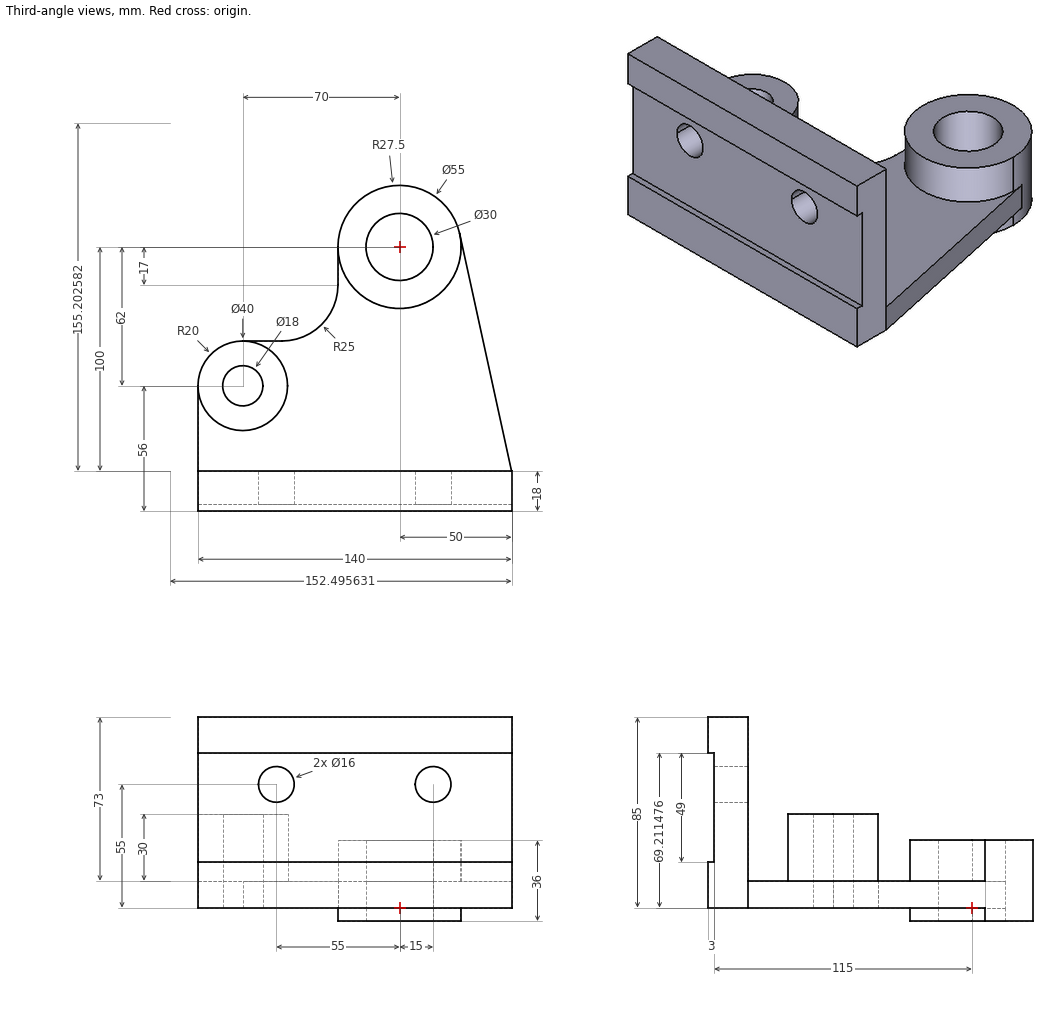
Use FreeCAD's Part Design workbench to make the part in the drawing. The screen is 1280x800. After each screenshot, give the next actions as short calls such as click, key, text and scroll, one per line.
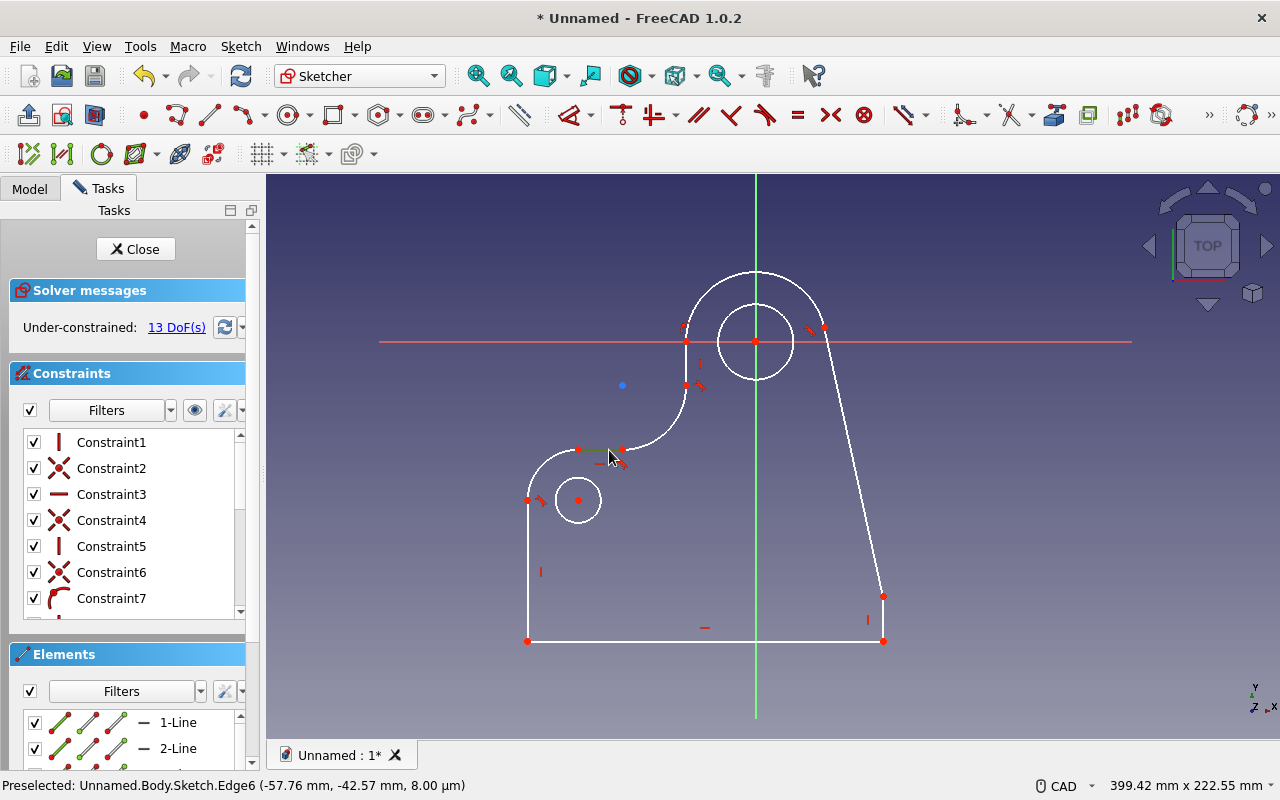
click(555, 455)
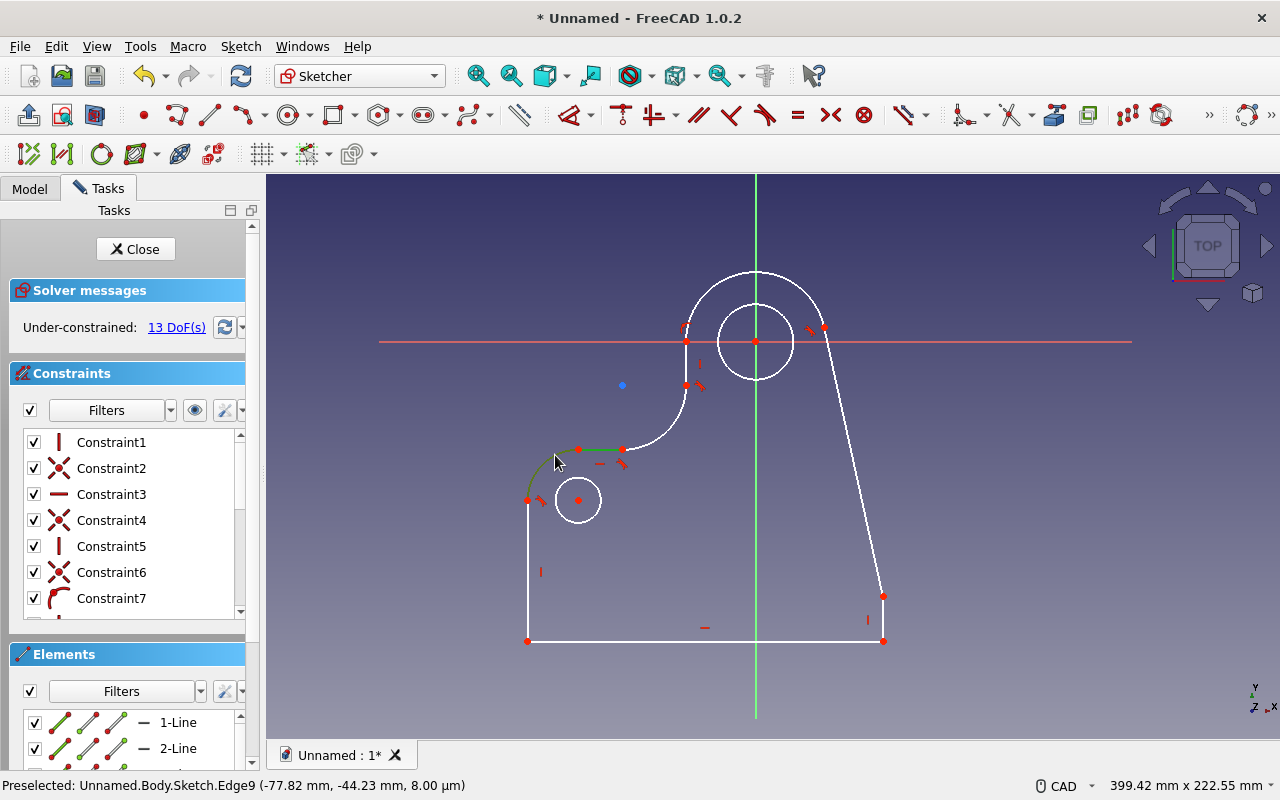
key(t)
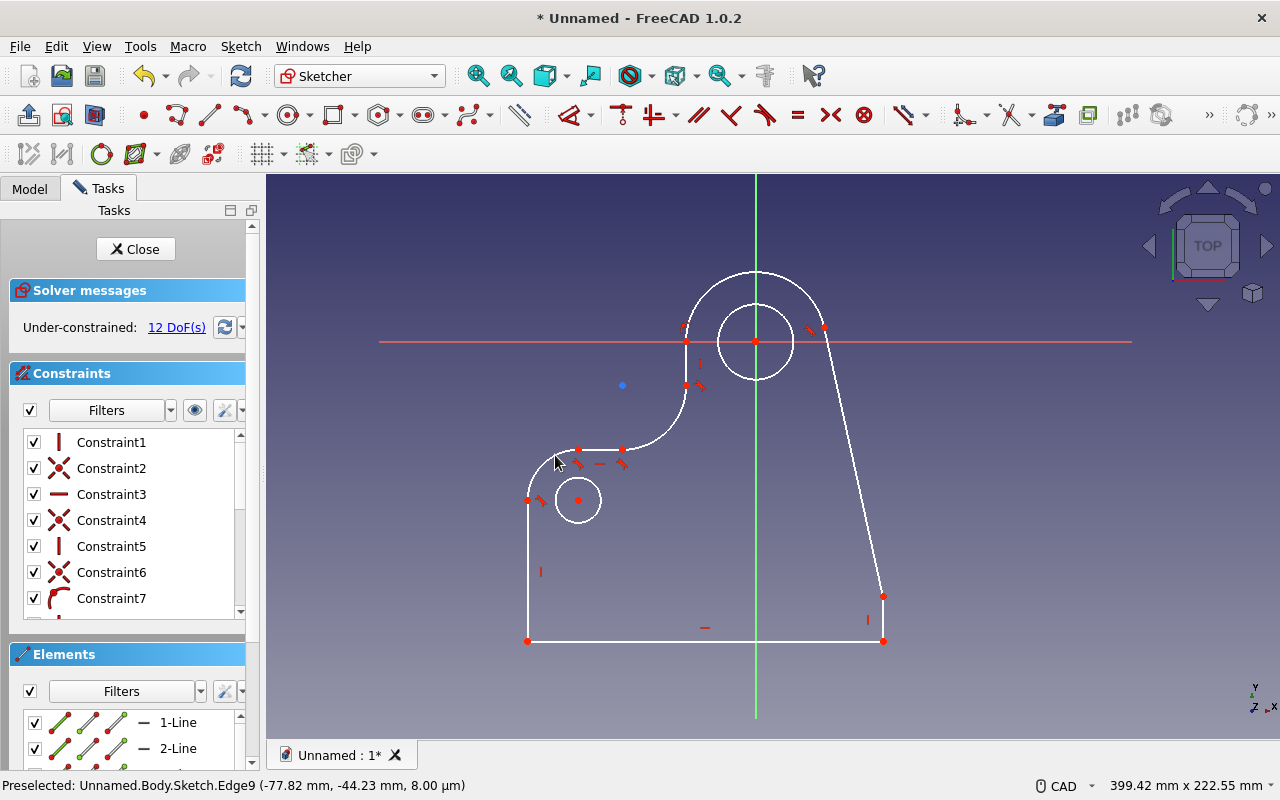
scroll(756, 342, up, 3)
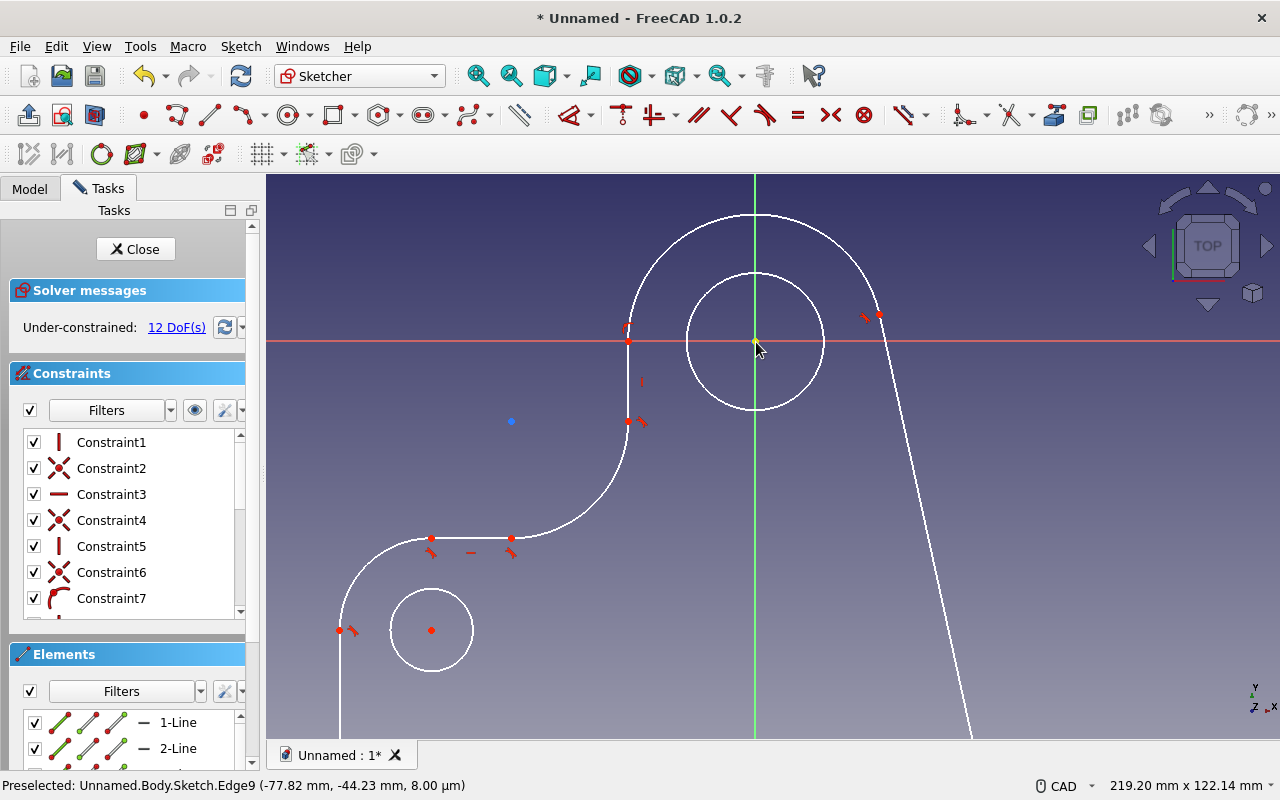
drag(745, 331, 765, 352)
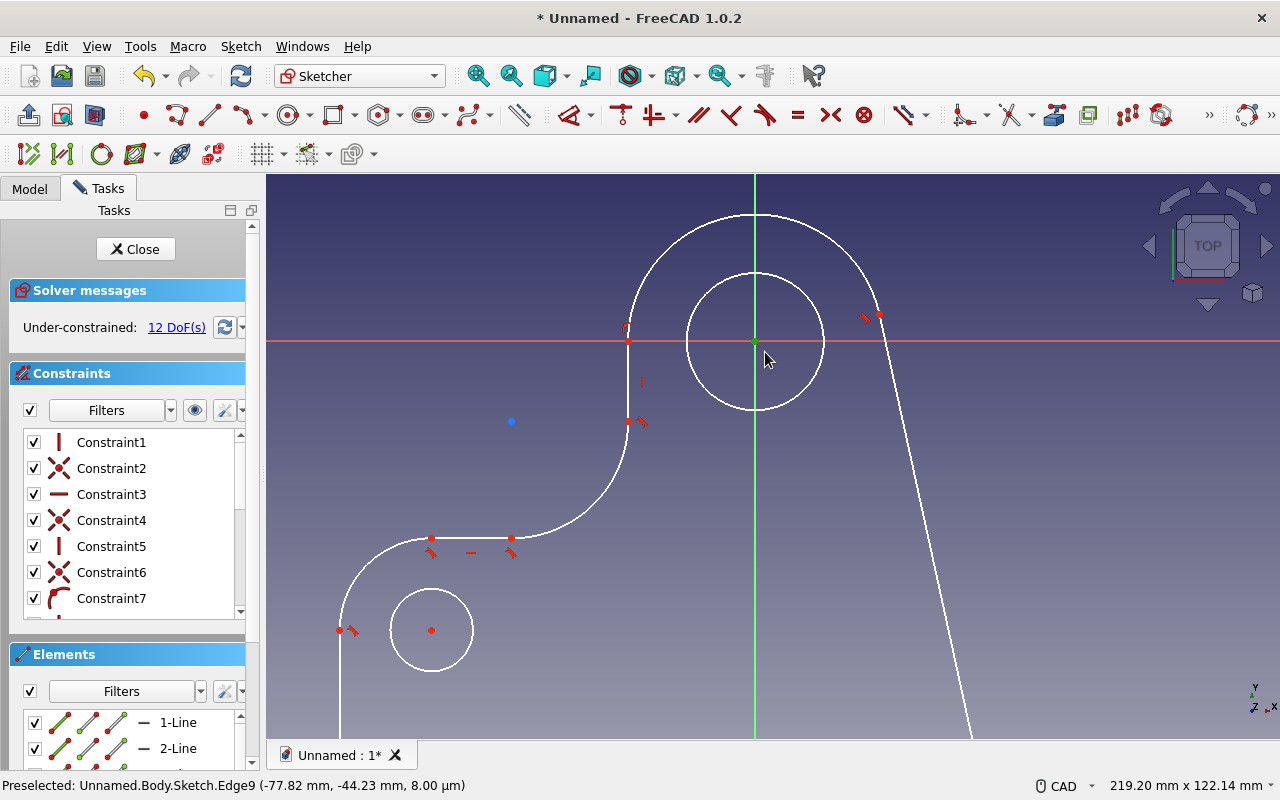
click(621, 116)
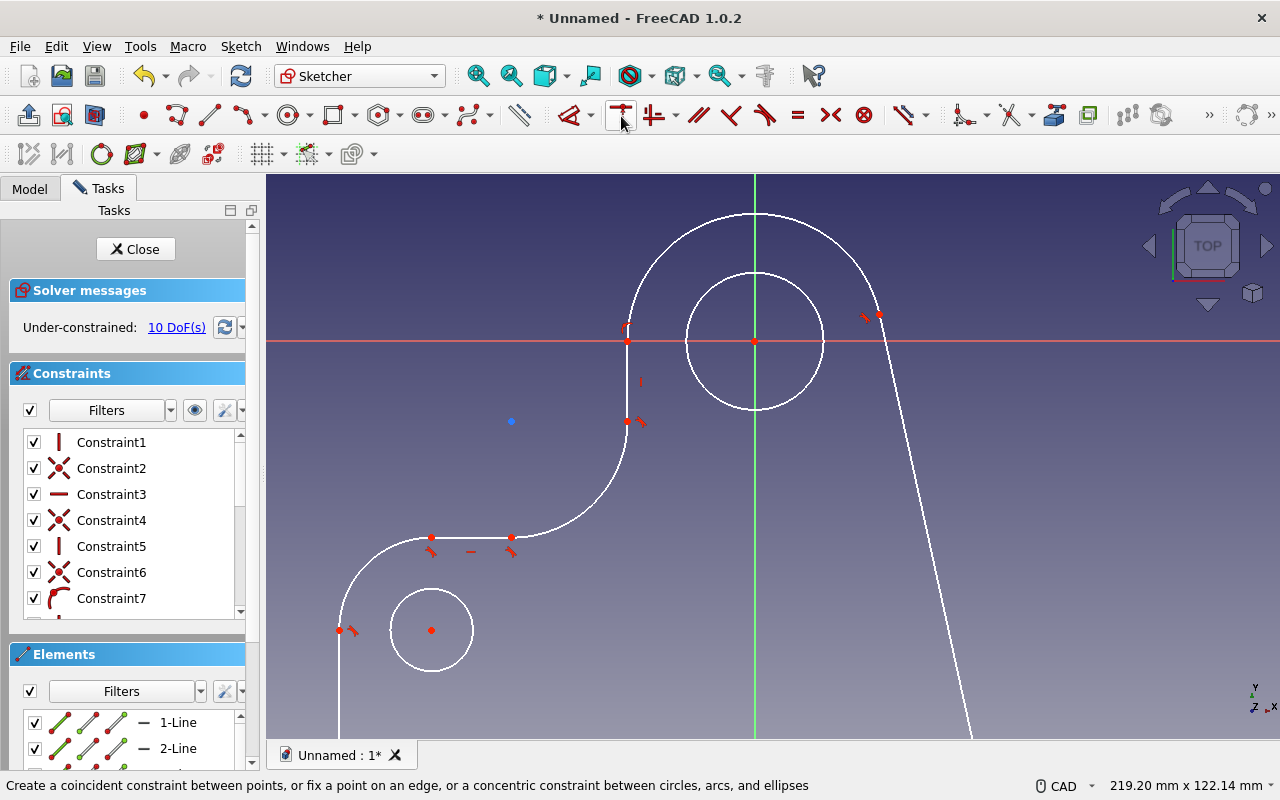
key(d)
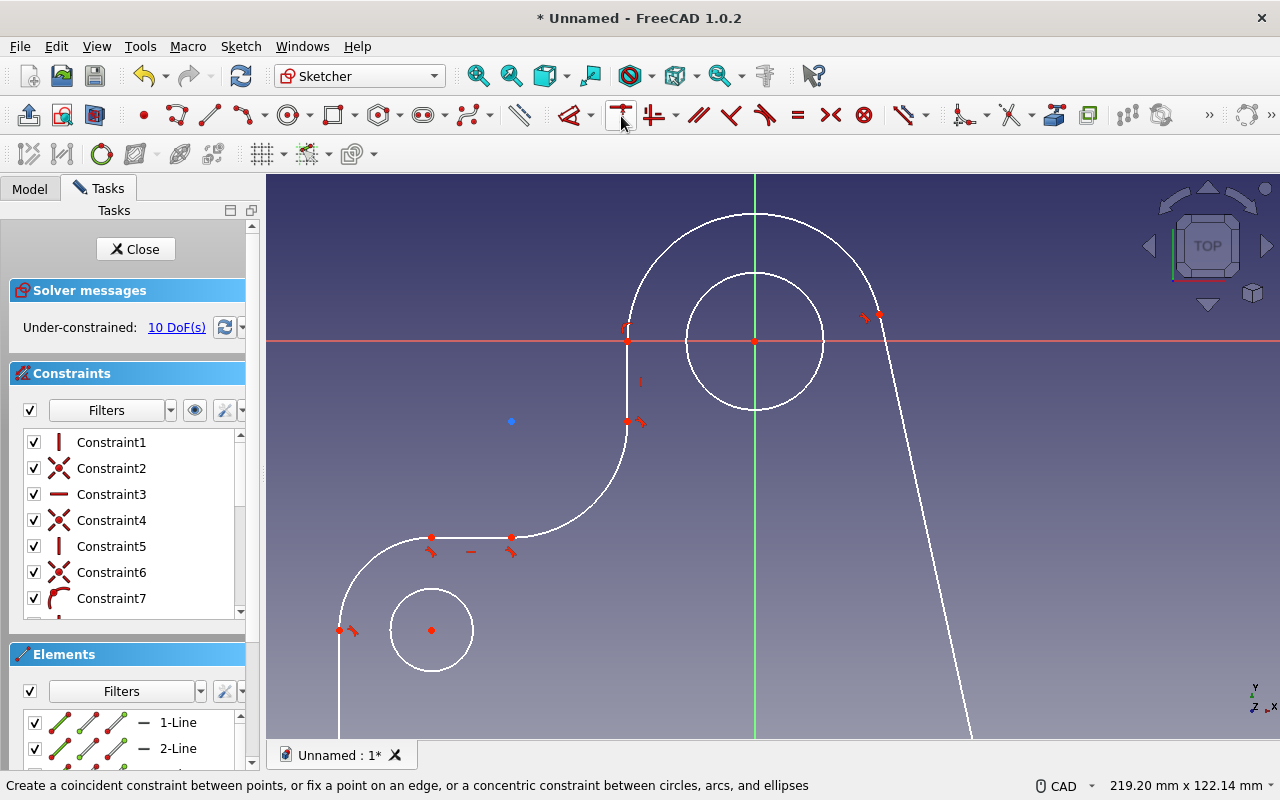
click(814, 228)
click(888, 252)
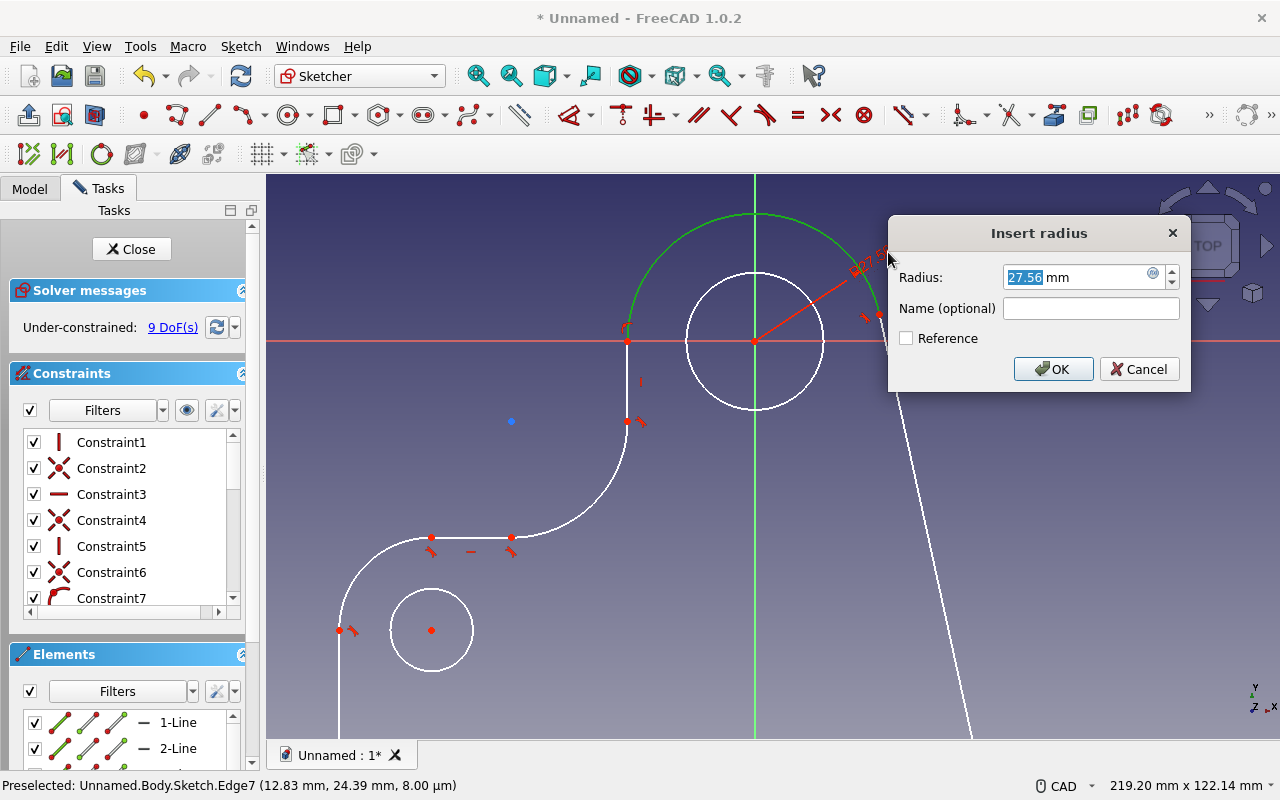
text(27.5)
key(Return)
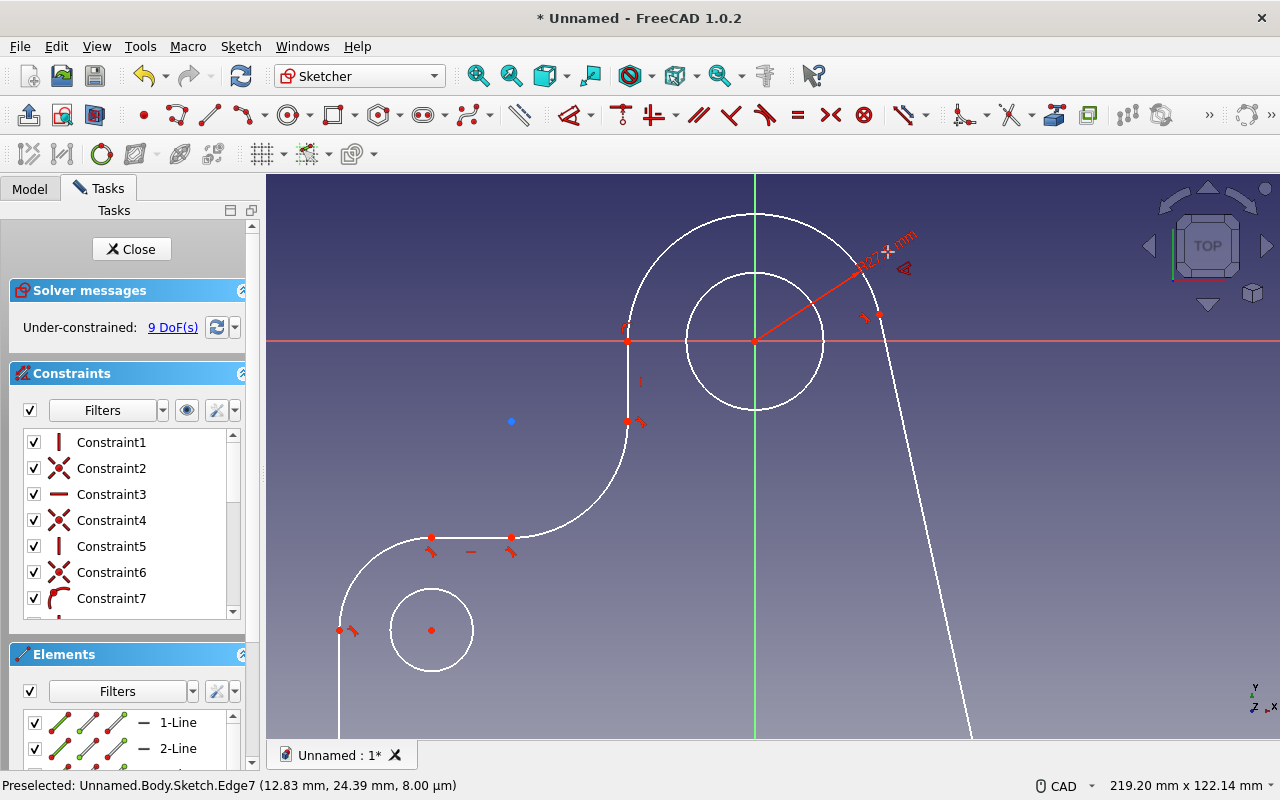
click(564, 525)
click(578, 554)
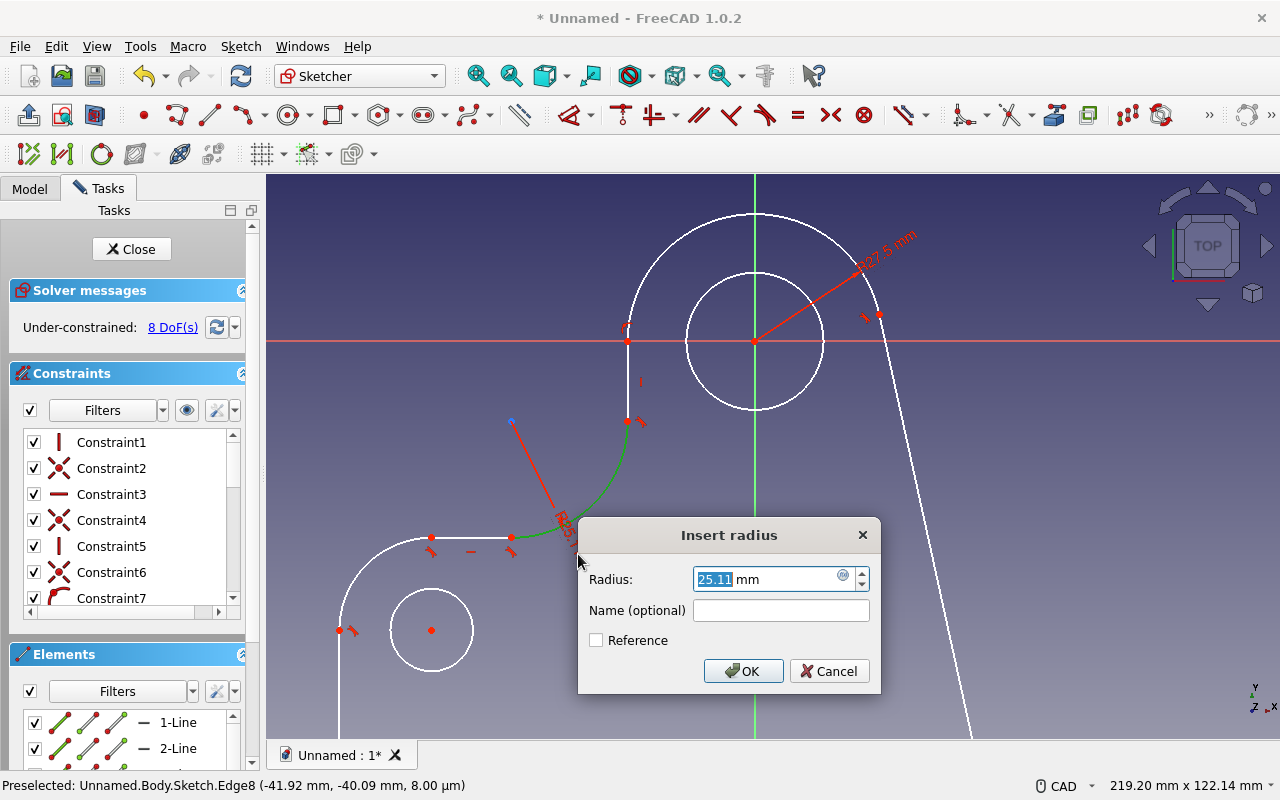
text(25)
key(Return)